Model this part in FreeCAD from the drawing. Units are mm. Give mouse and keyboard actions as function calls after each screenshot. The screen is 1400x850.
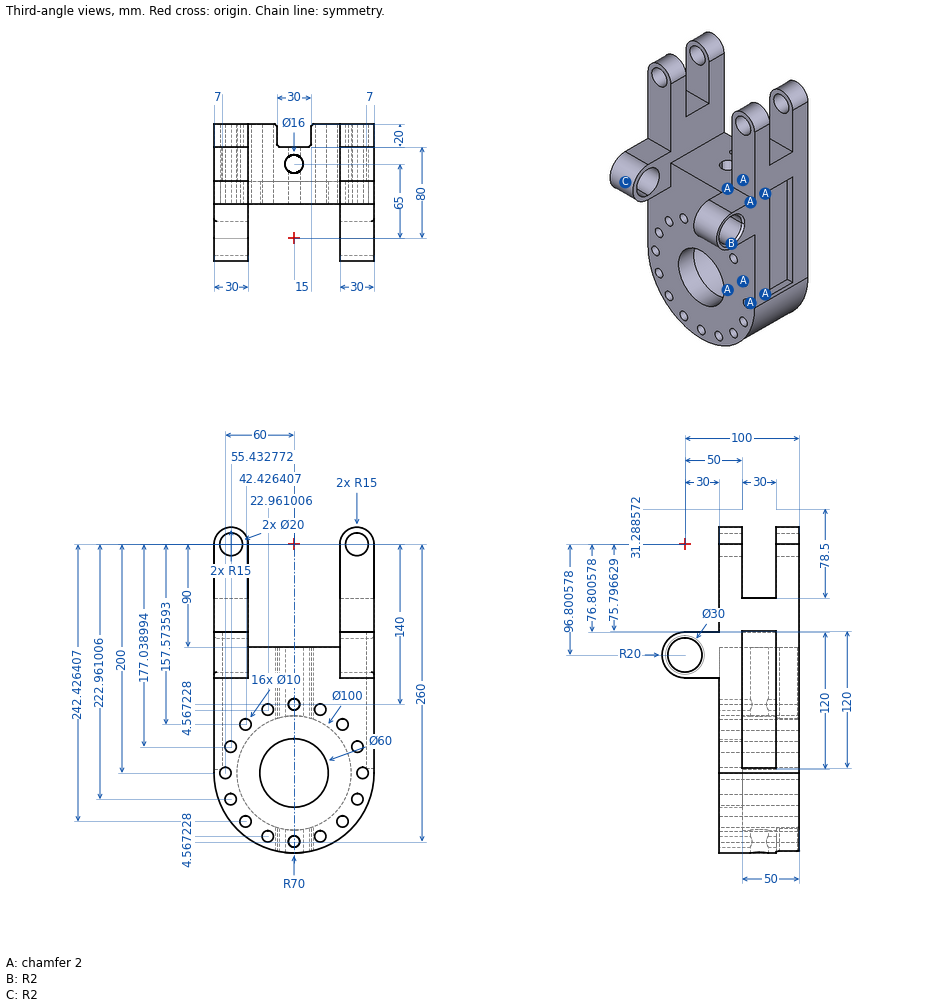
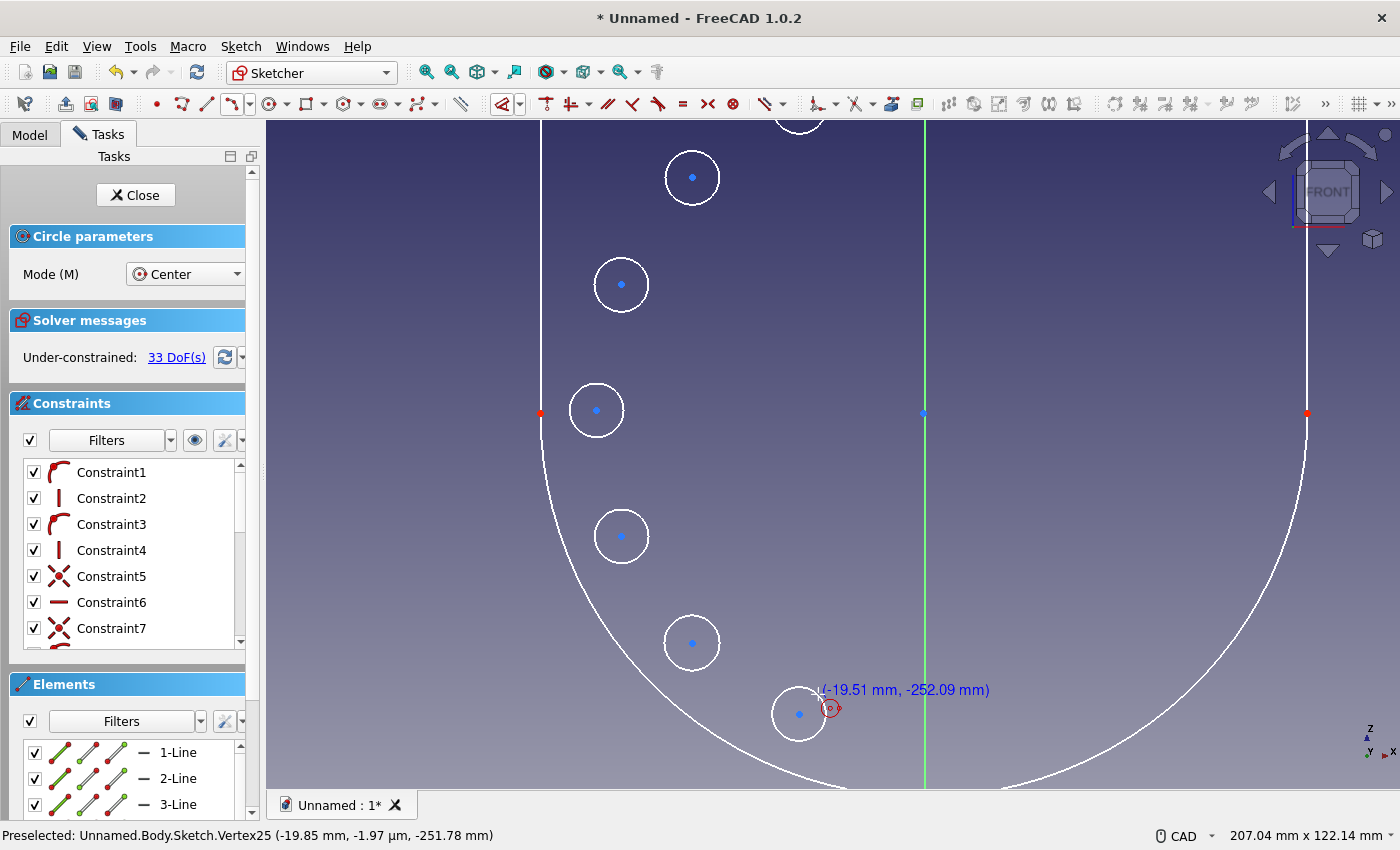
scroll(695, 645, down, 6)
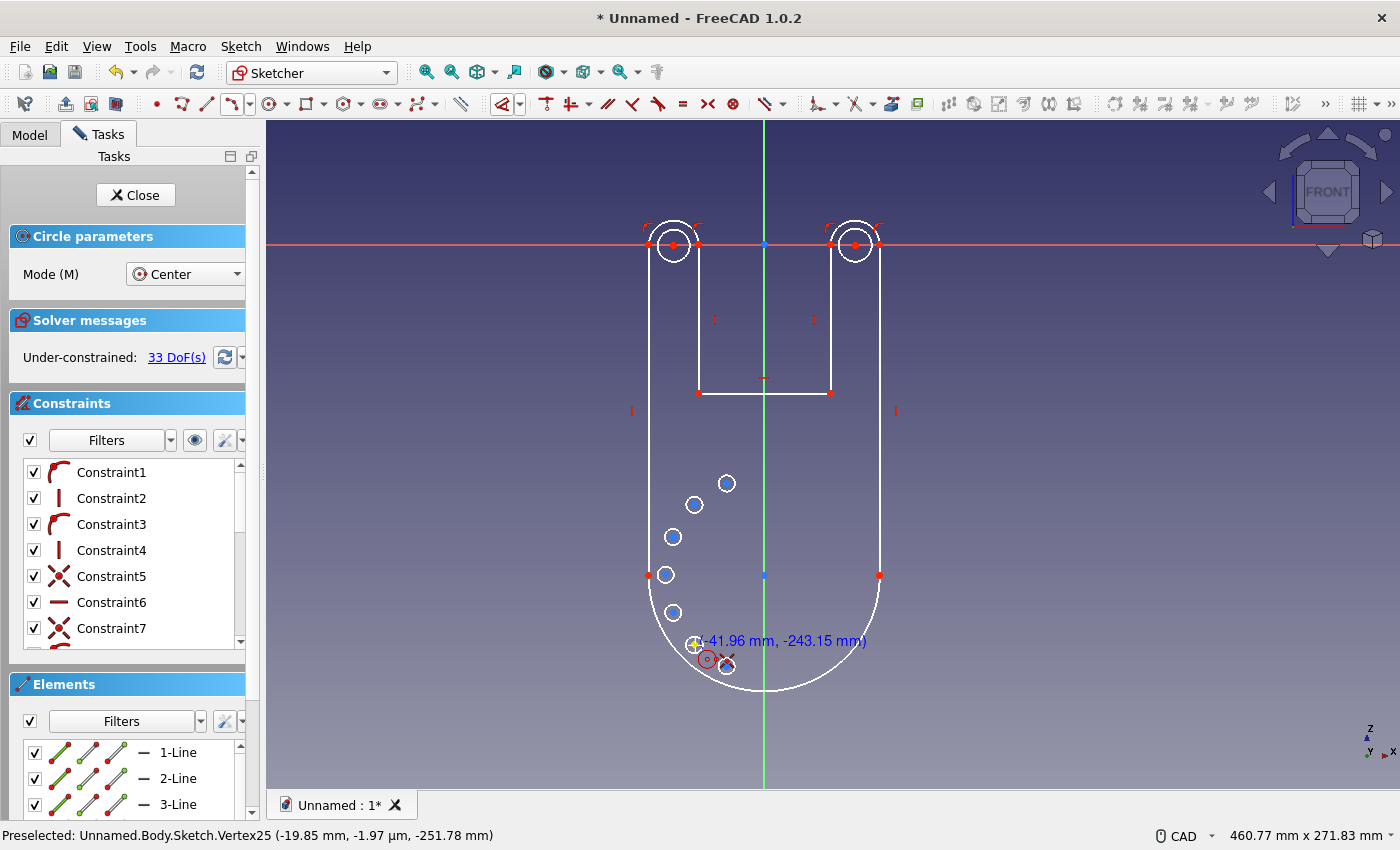
scroll(764, 476, up, 6)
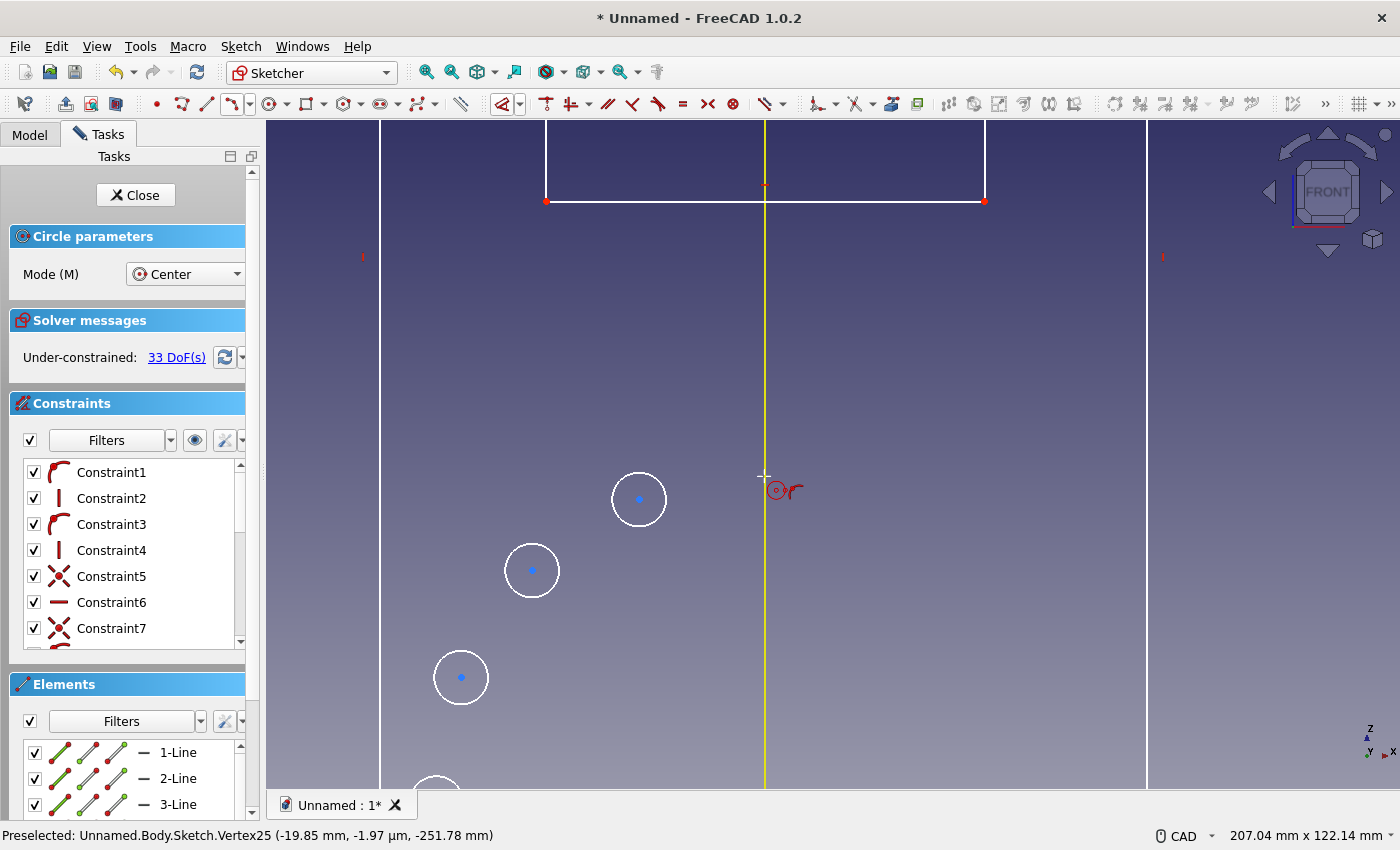
click(765, 474)
click(784, 454)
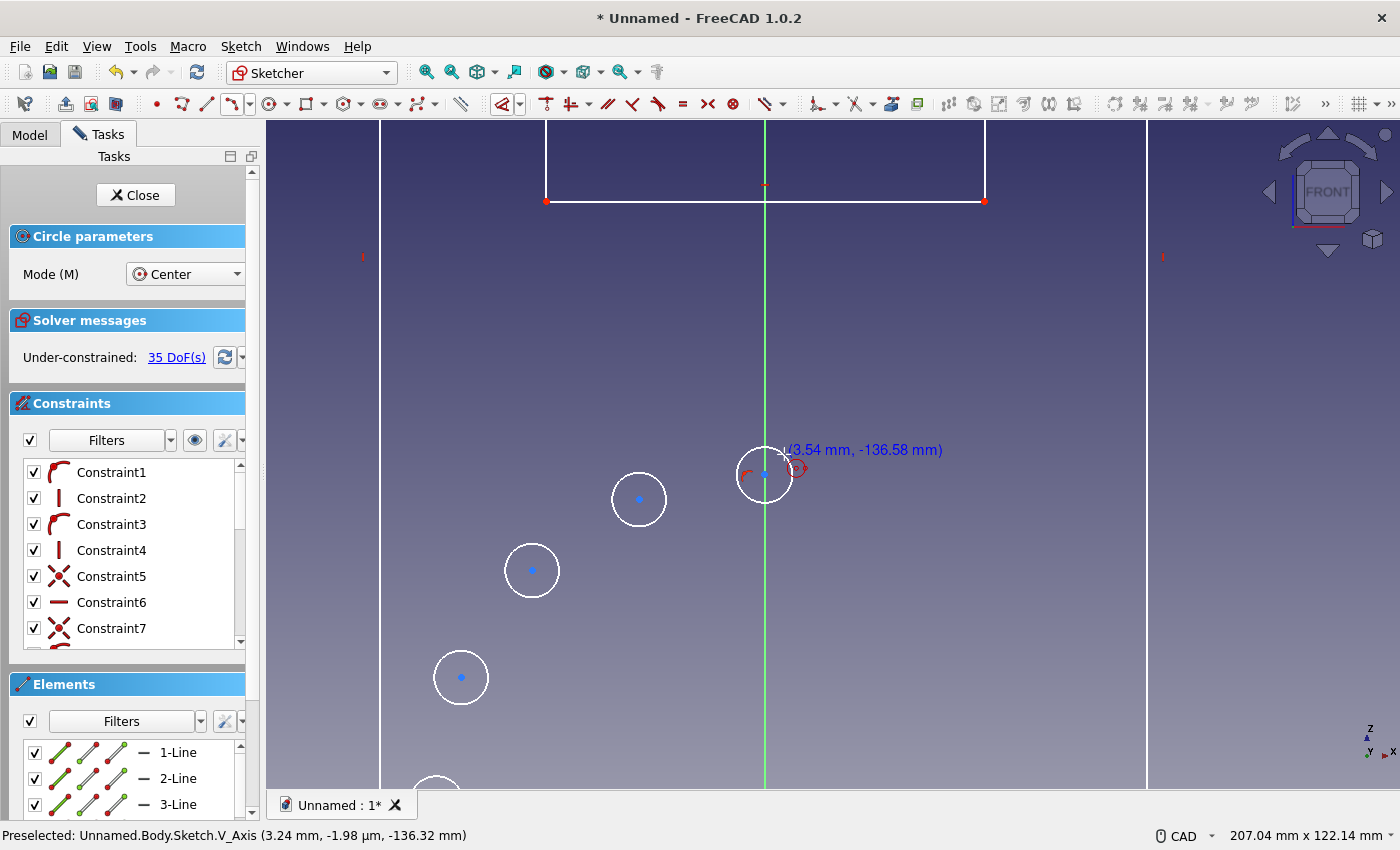
click(890, 499)
click(910, 479)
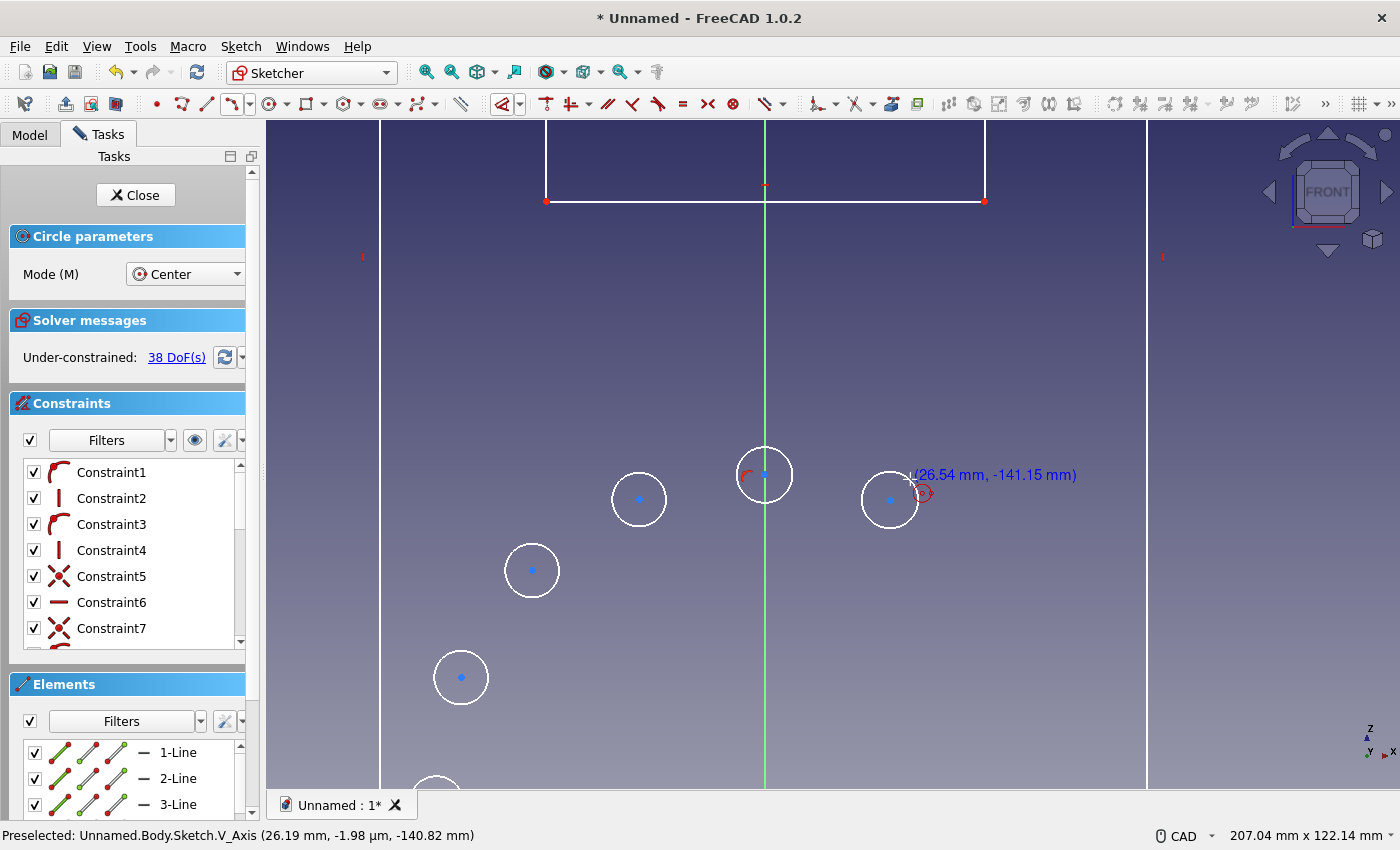
click(997, 570)
click(1016, 551)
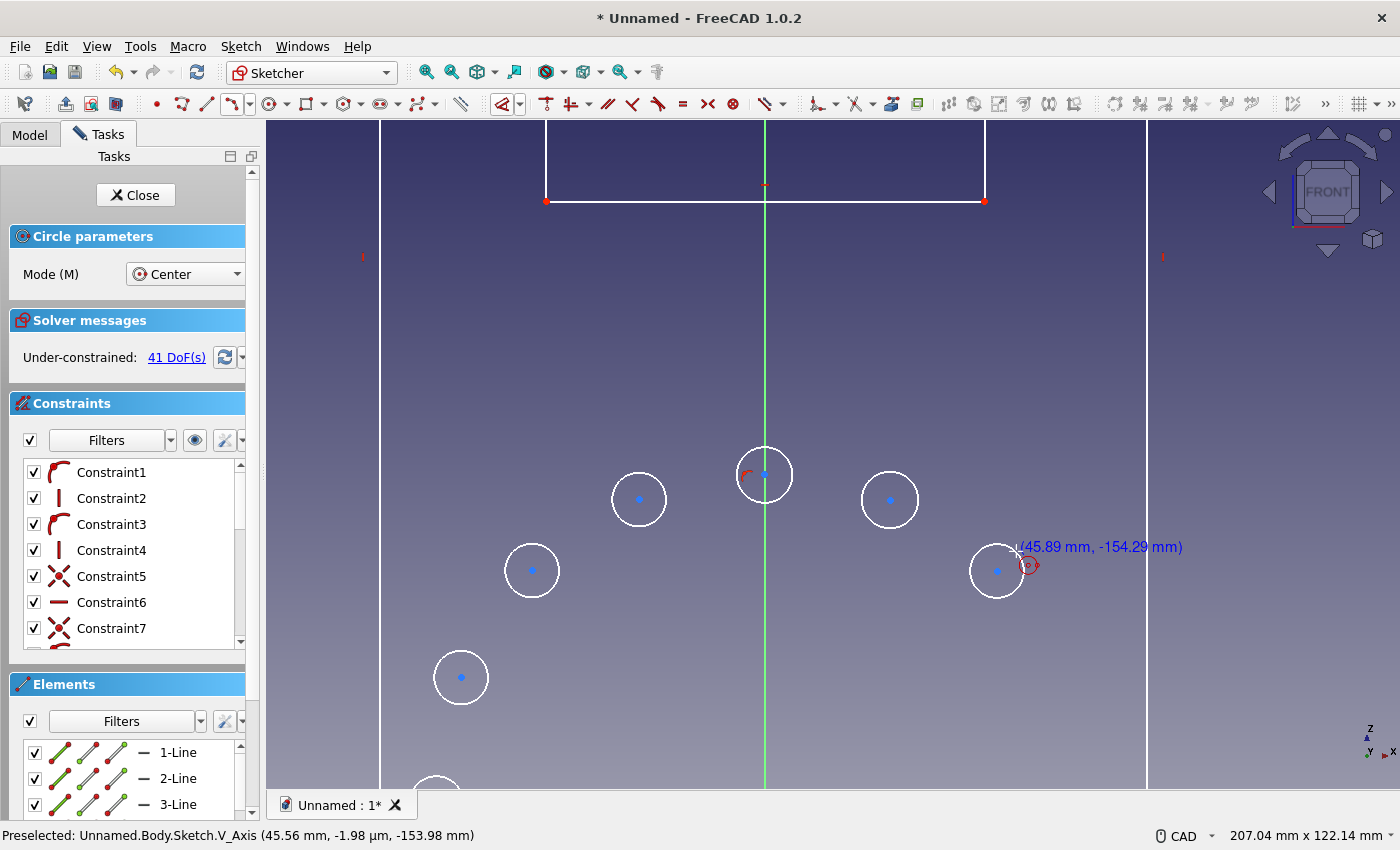
click(1068, 677)
click(1088, 657)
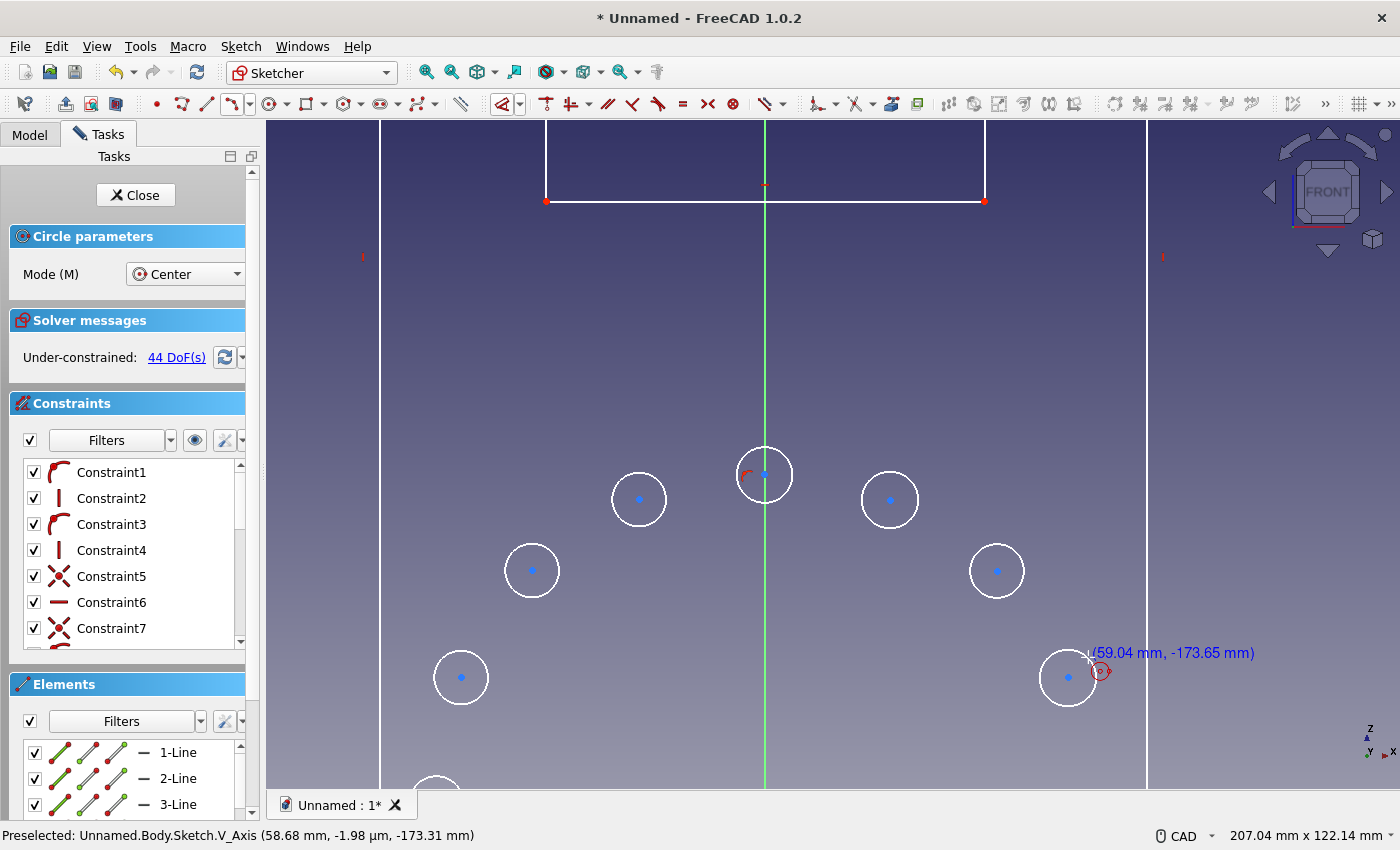
scroll(764, 476, down, 6)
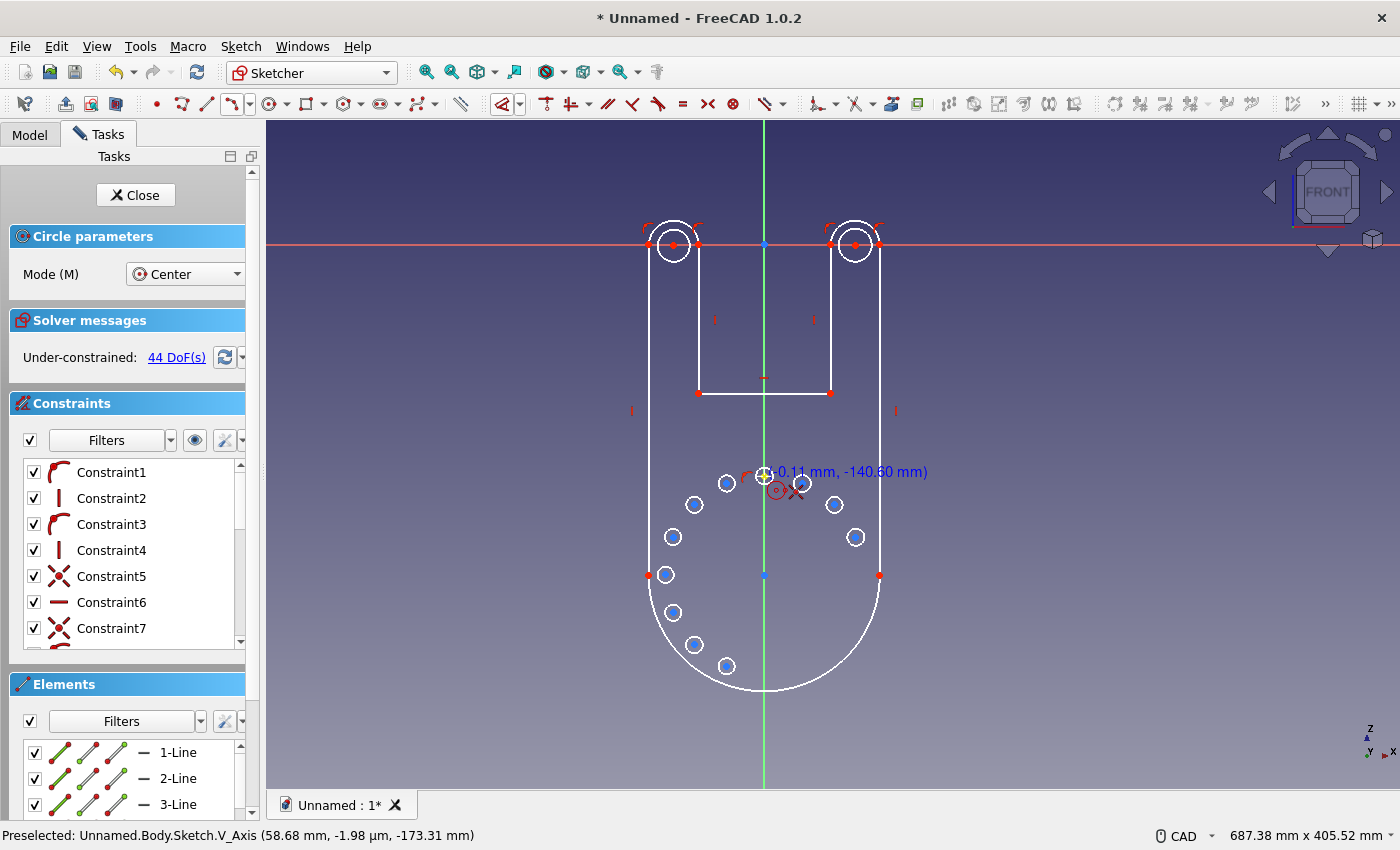
click(764, 575)
click(799, 540)